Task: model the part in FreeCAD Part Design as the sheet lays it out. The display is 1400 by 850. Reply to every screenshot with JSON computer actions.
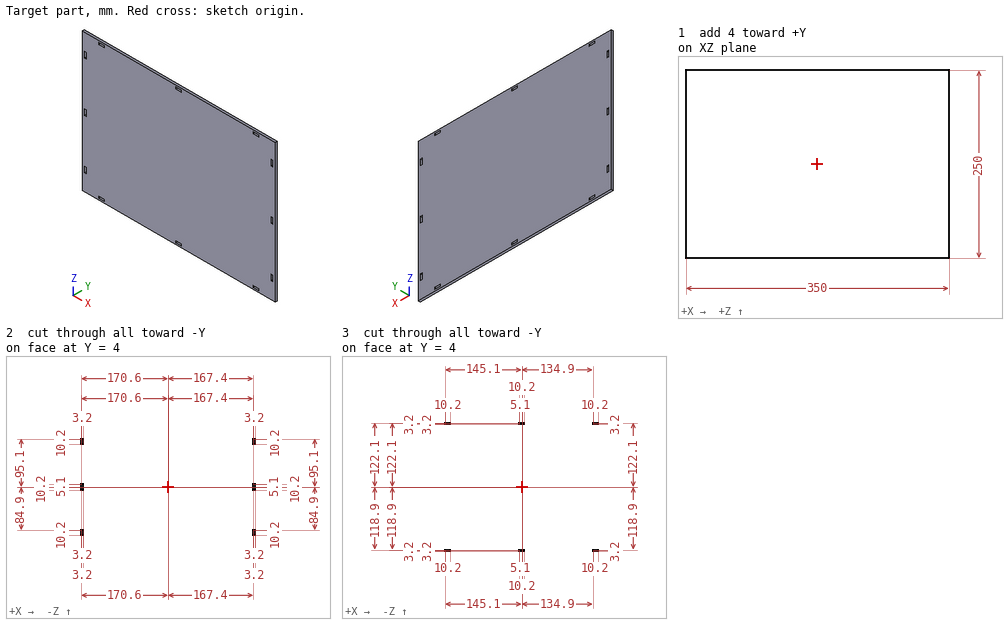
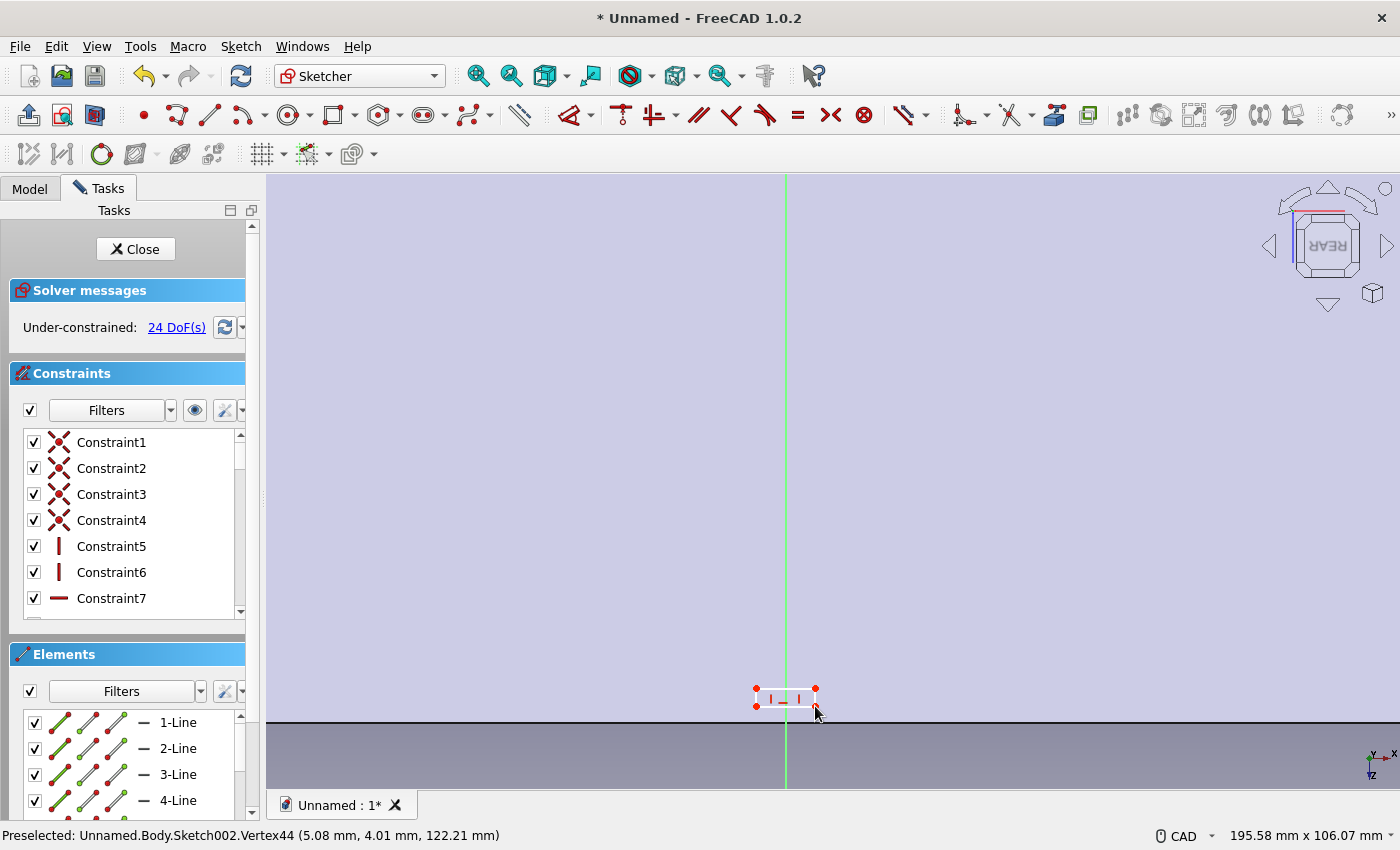
{"action": "left_click", "coordinate": [568, 116]}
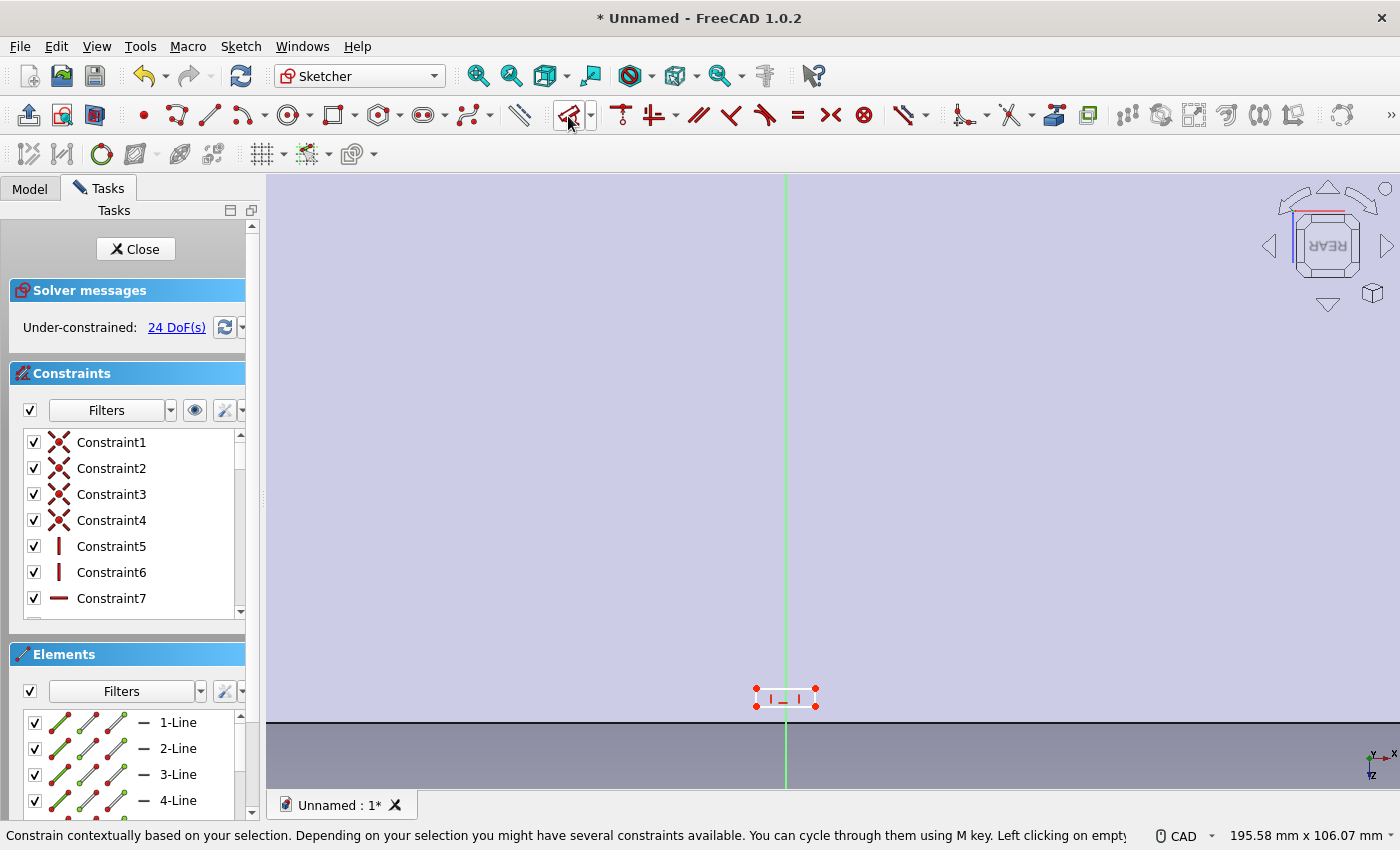
{"action": "scroll", "coordinate": [755, 690], "scroll_direction": "down", "scroll_amount": 6}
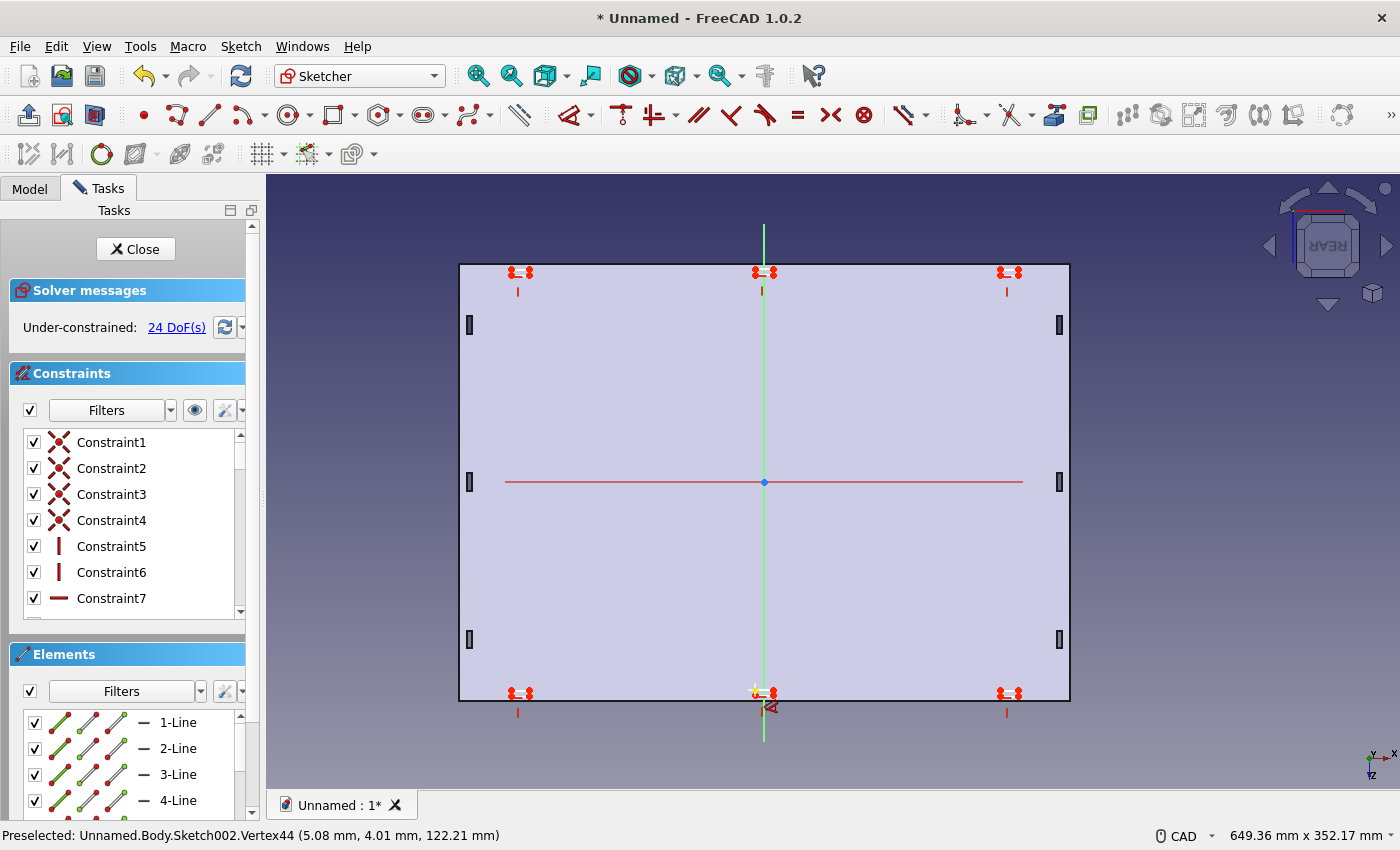
{"action": "scroll", "coordinate": [755, 272], "scroll_direction": "up", "scroll_amount": 10}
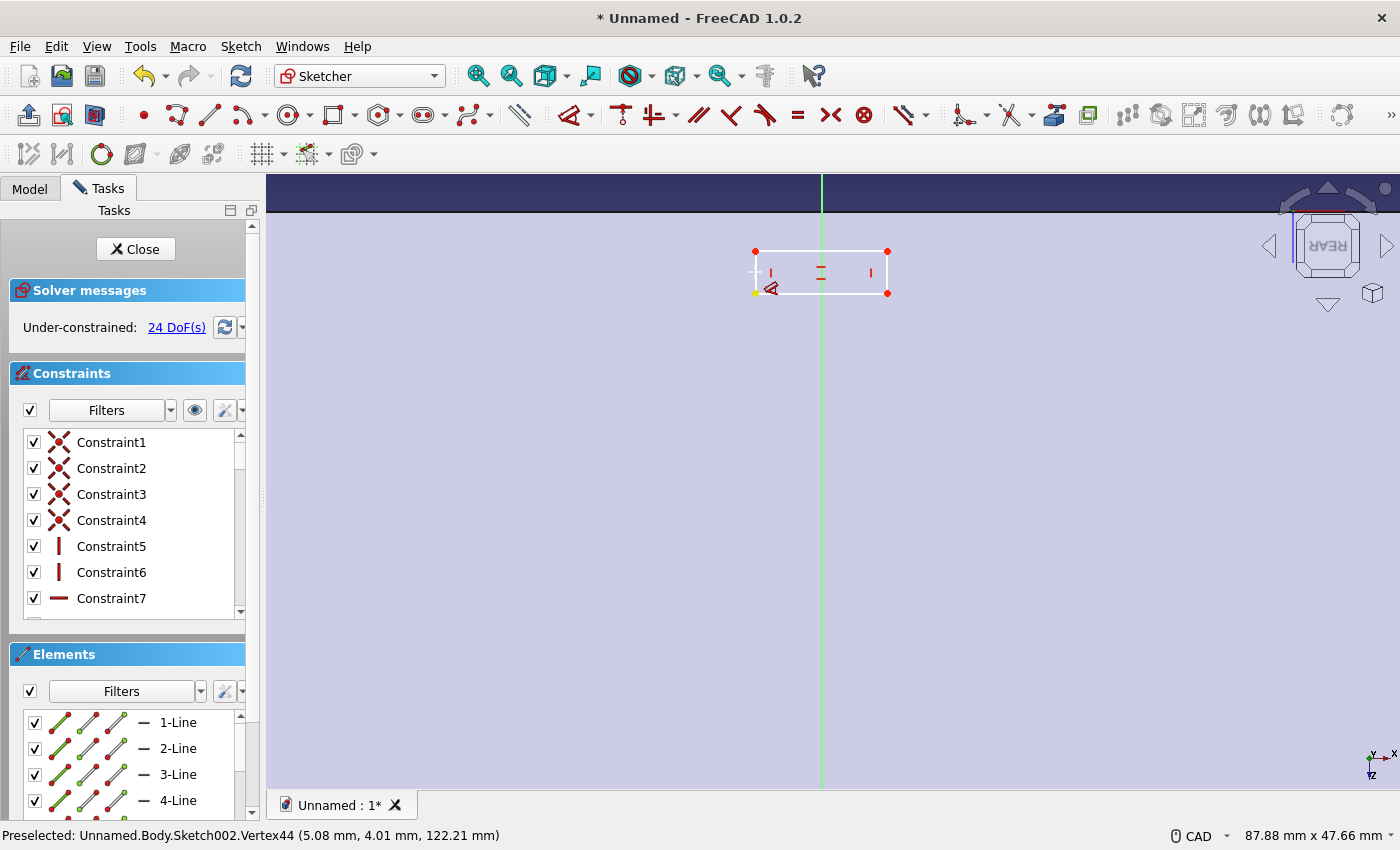
{"action": "left_click", "coordinate": [756, 273]}
{"action": "left_click", "coordinate": [722, 273]}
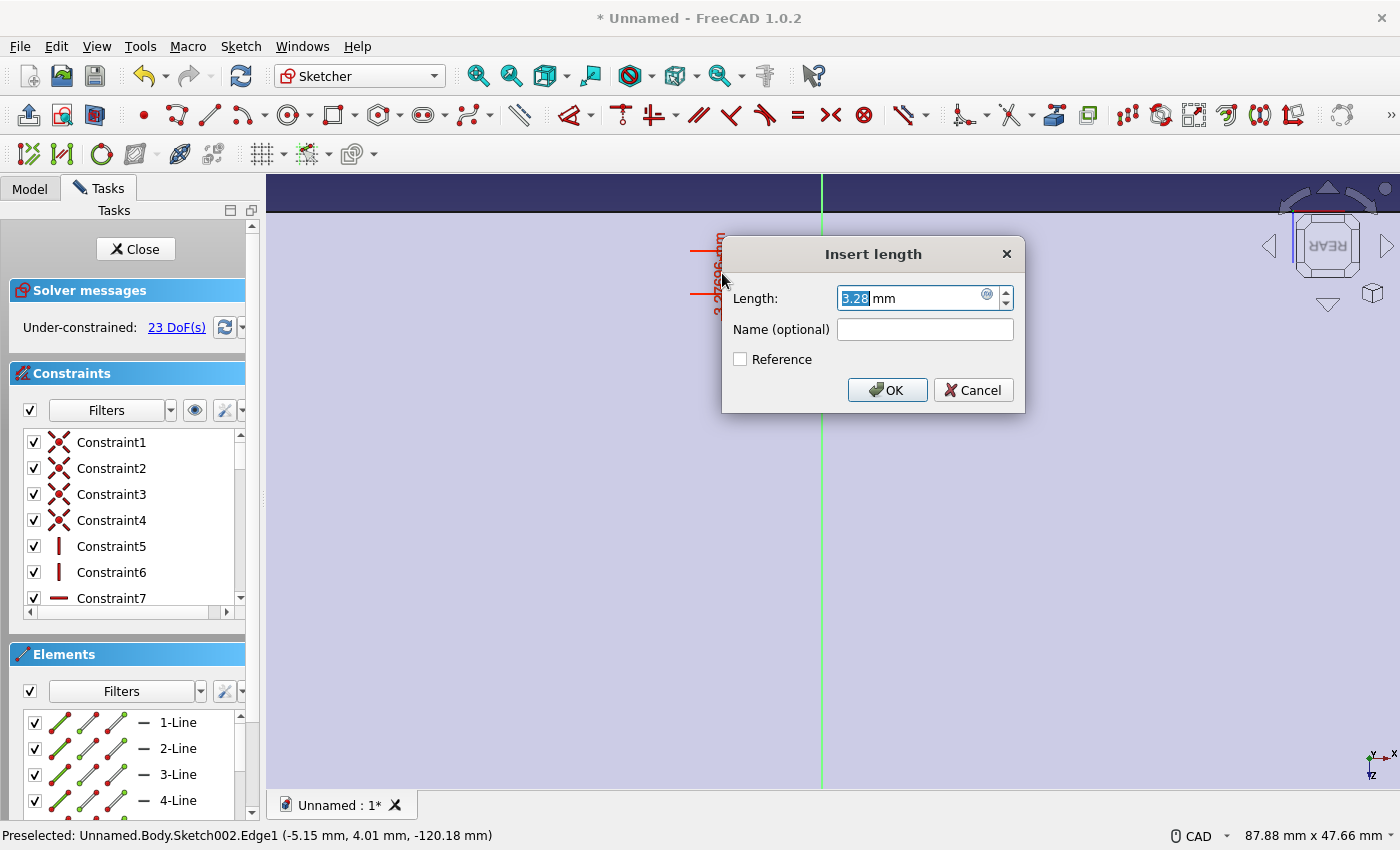
{"action": "type", "text": "3.2"}
{"action": "key", "text": "Return"}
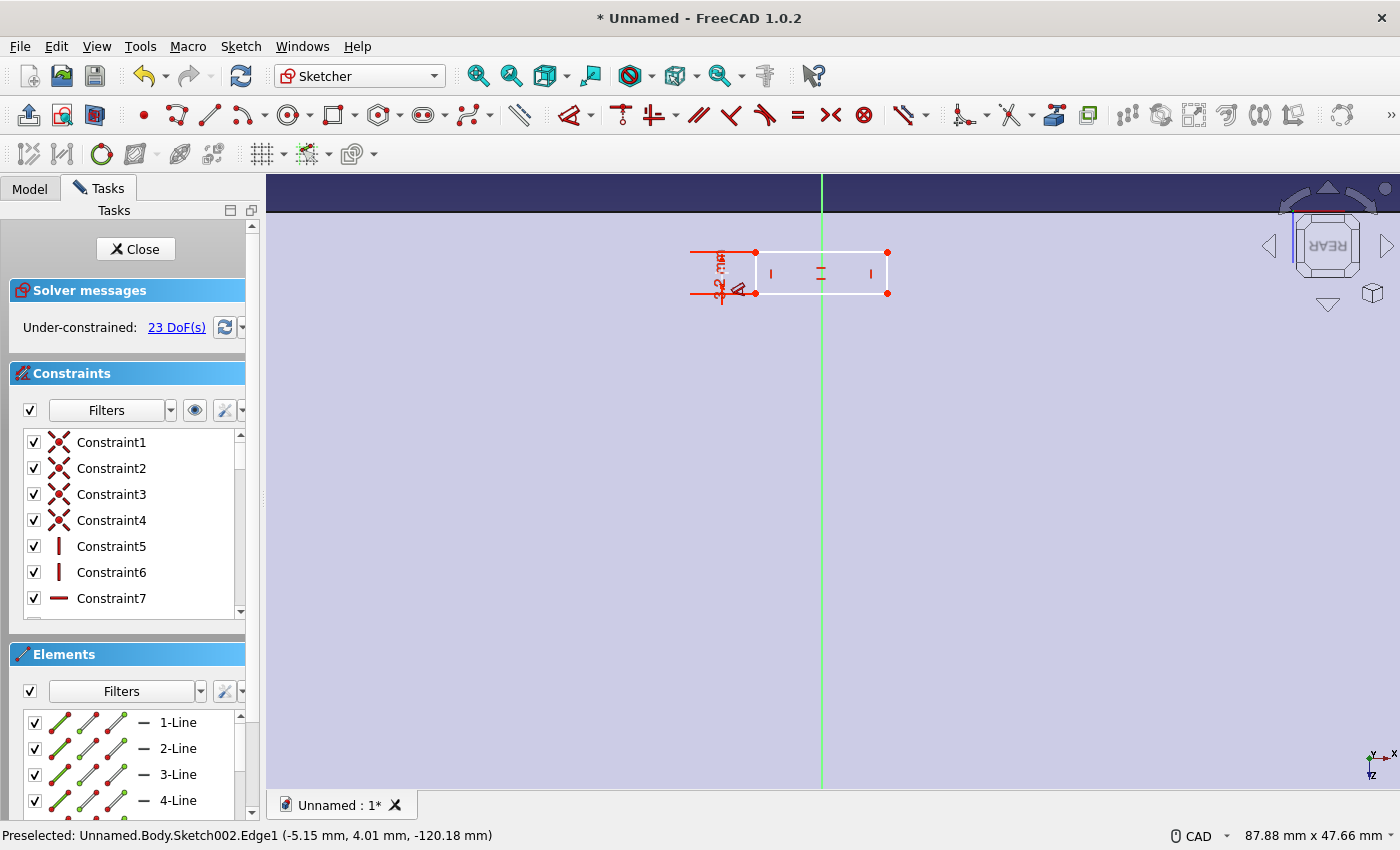
{"action": "scroll", "coordinate": [755, 271], "scroll_direction": "down", "scroll_amount": 10}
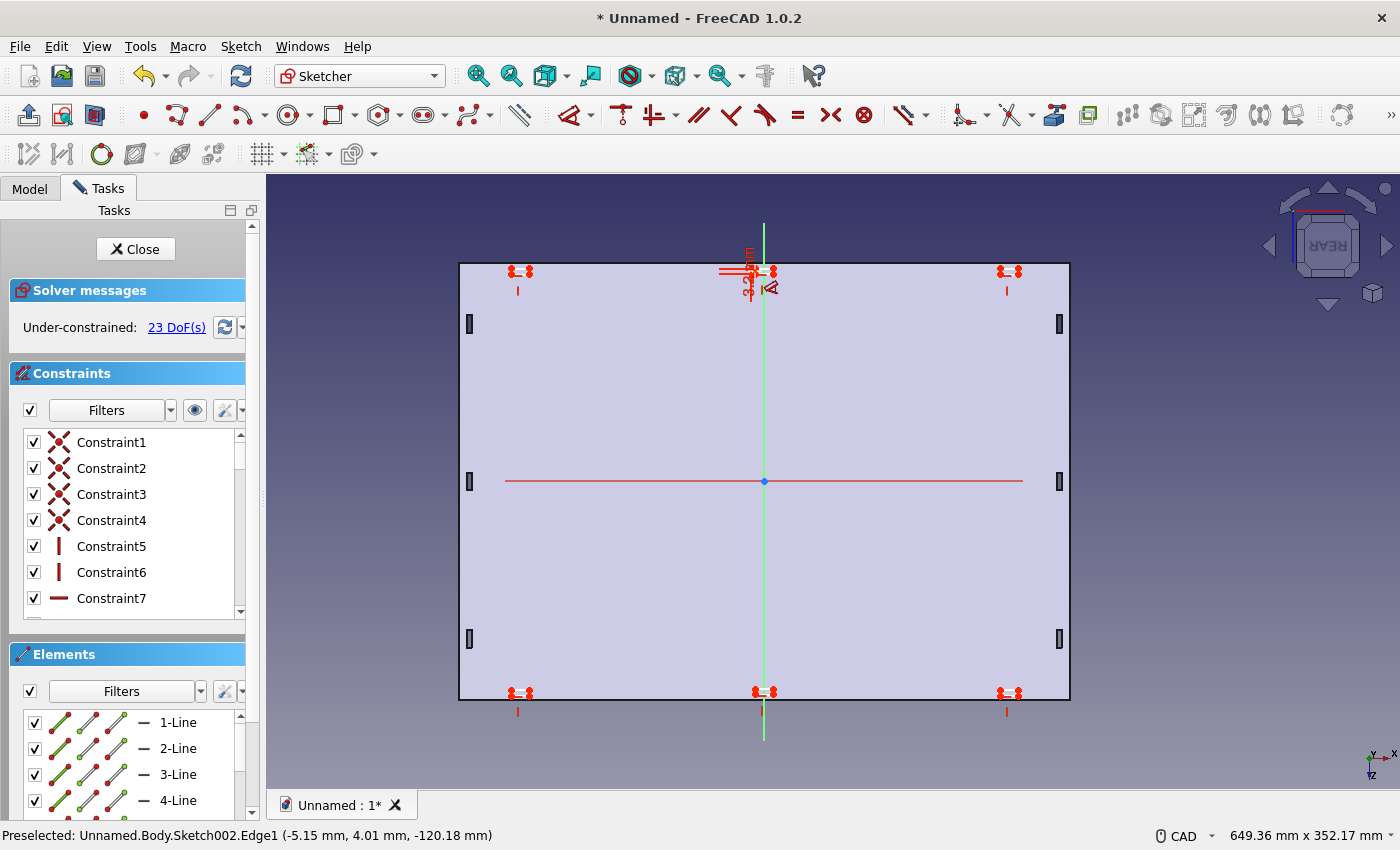
{"action": "scroll", "coordinate": [1000, 271], "scroll_direction": "up", "scroll_amount": 11}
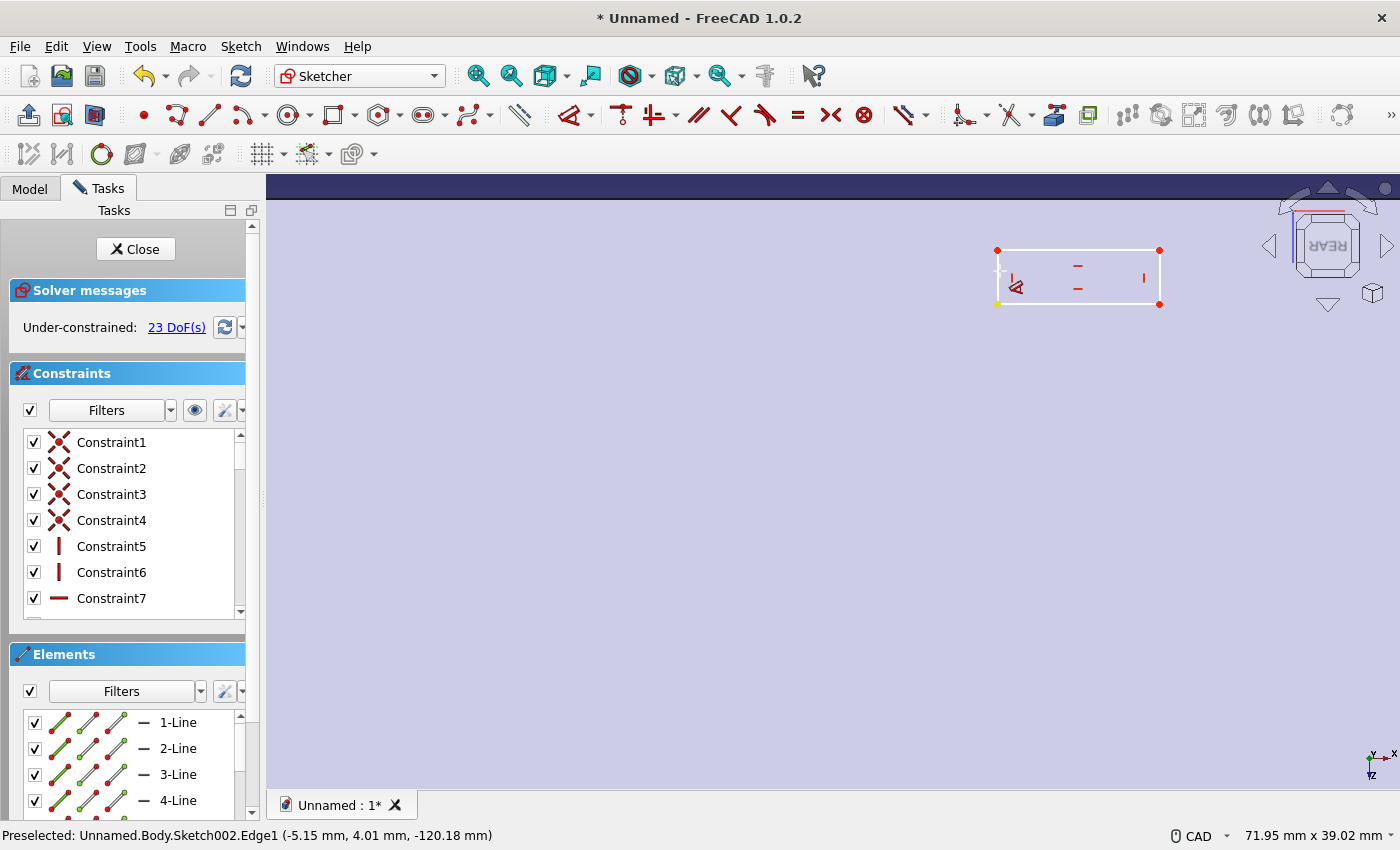
{"action": "left_click", "coordinate": [998, 266]}
{"action": "left_click", "coordinate": [1032, 277]}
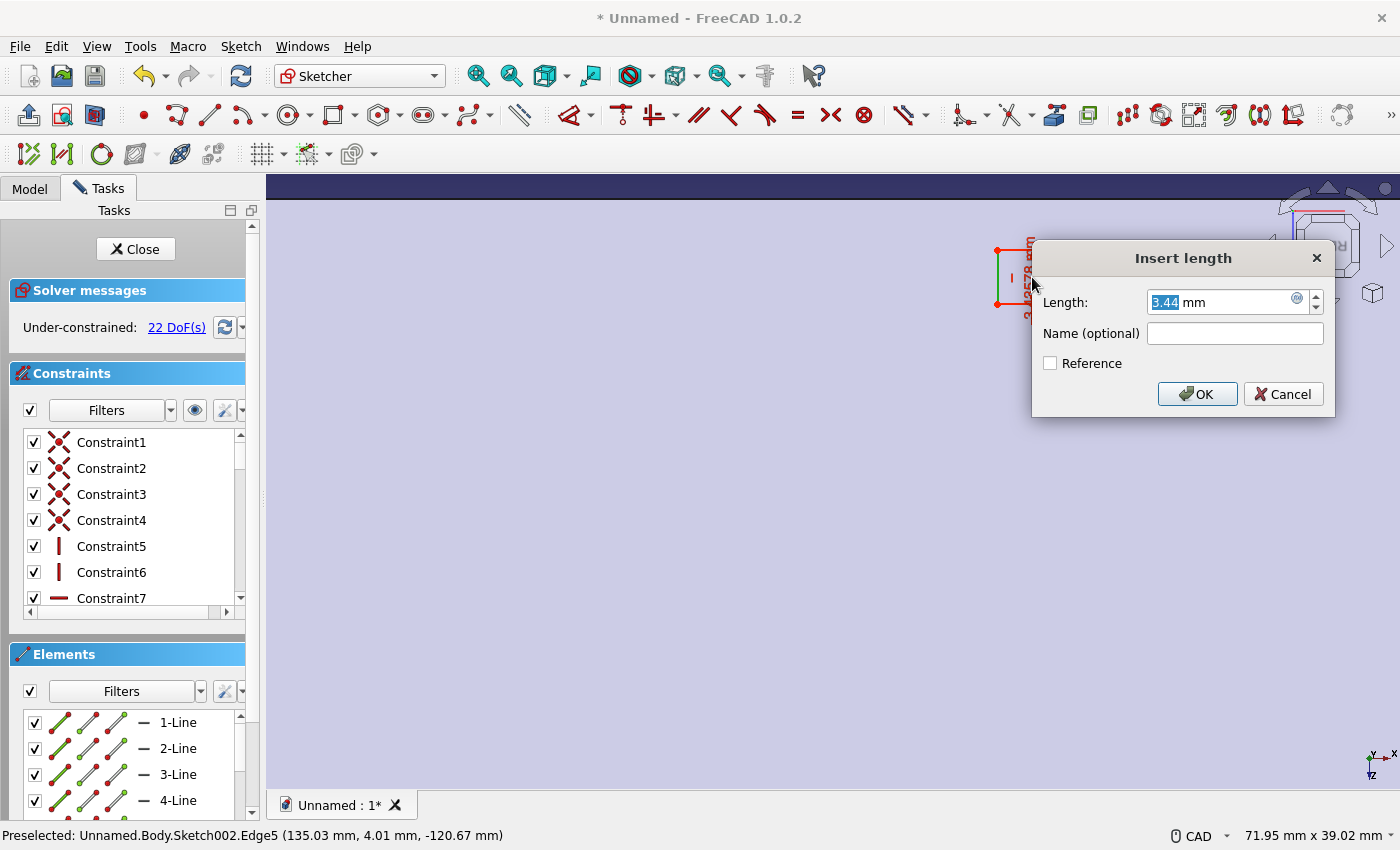
{"action": "type", "text": "3.2"}
{"action": "key", "text": "Return"}